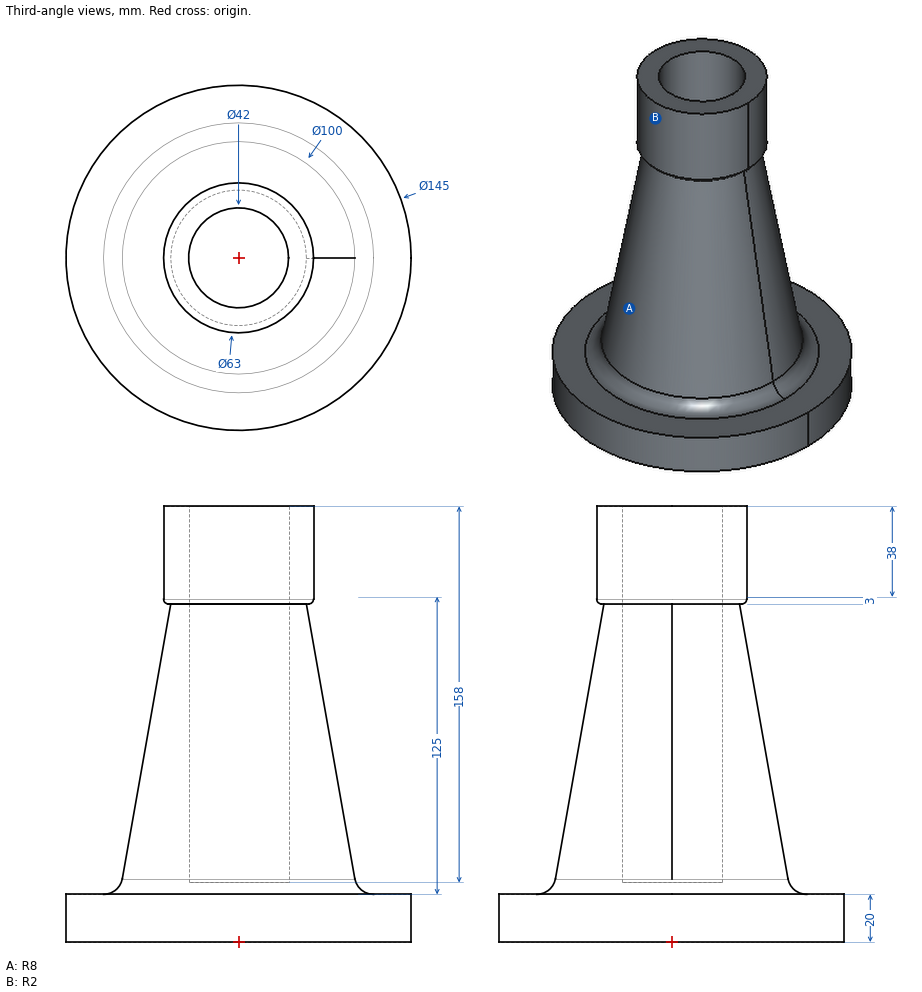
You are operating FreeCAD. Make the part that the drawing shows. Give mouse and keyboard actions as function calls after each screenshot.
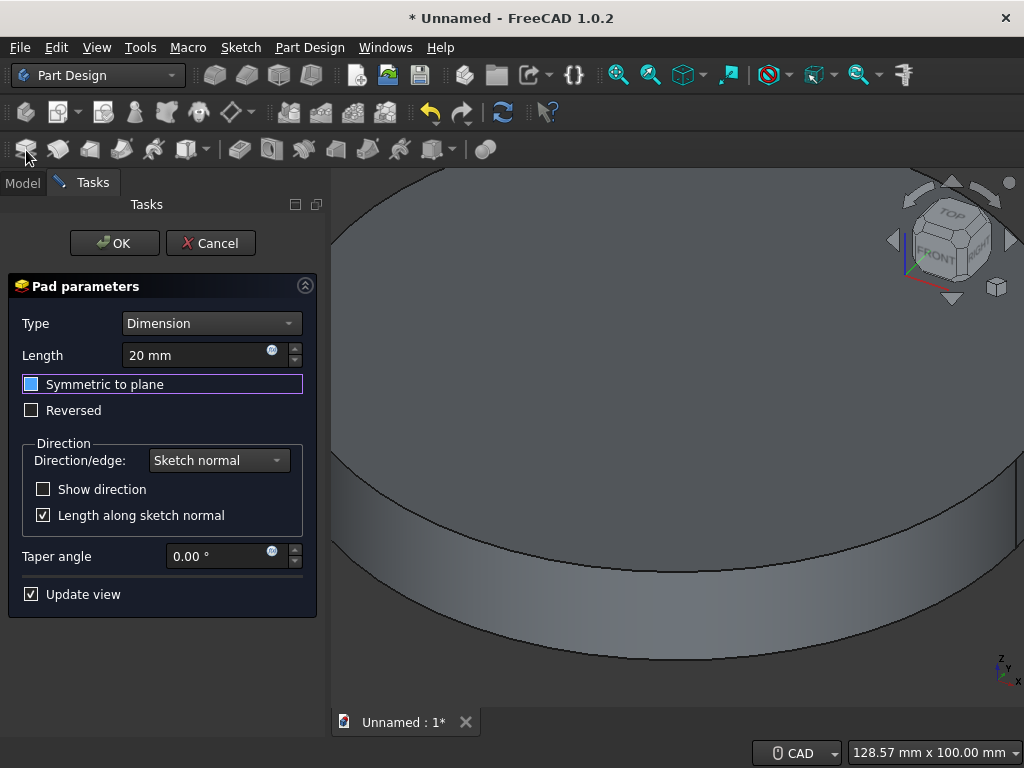
click(115, 243)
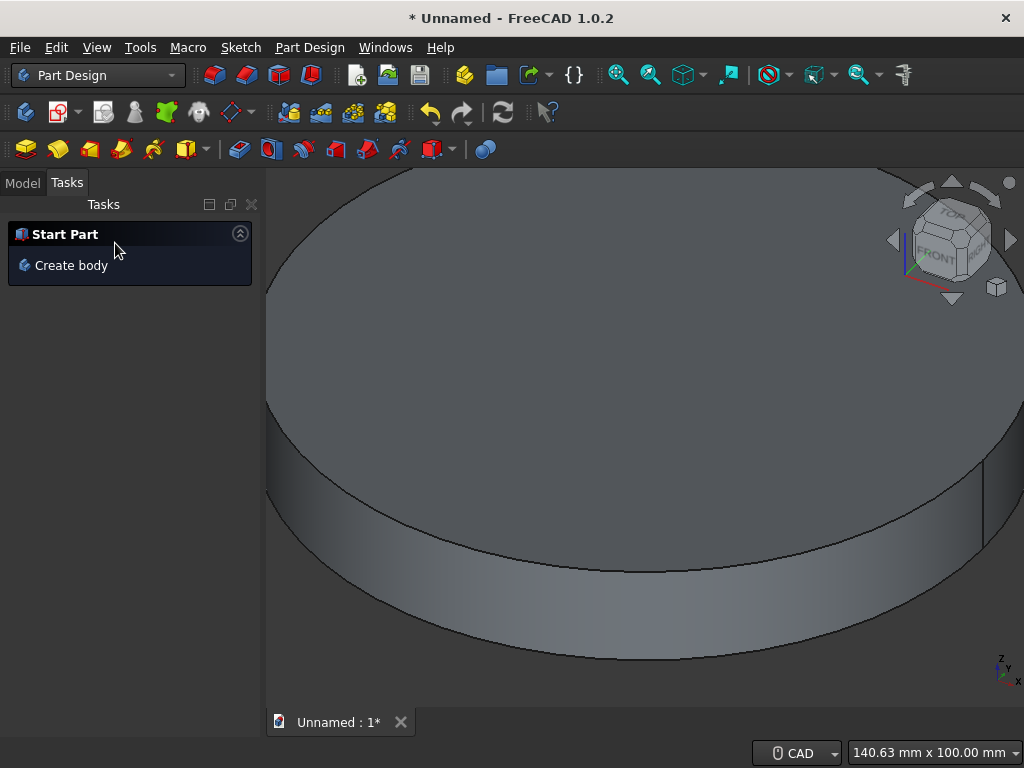
key(v)
key(f)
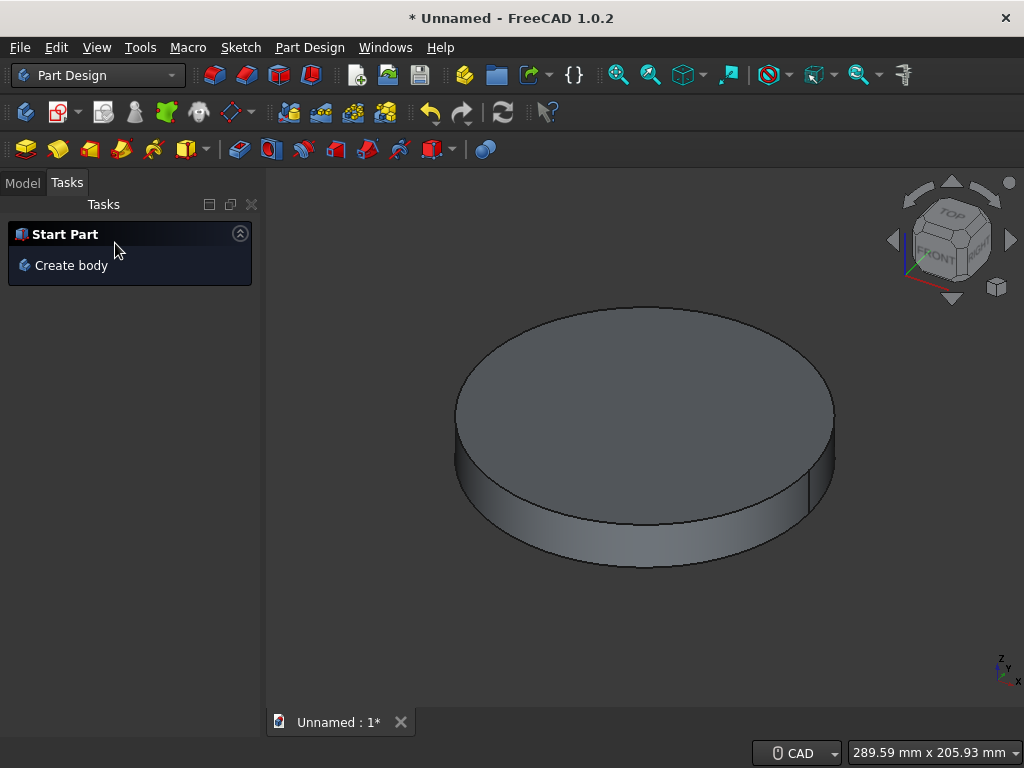
click(645, 415)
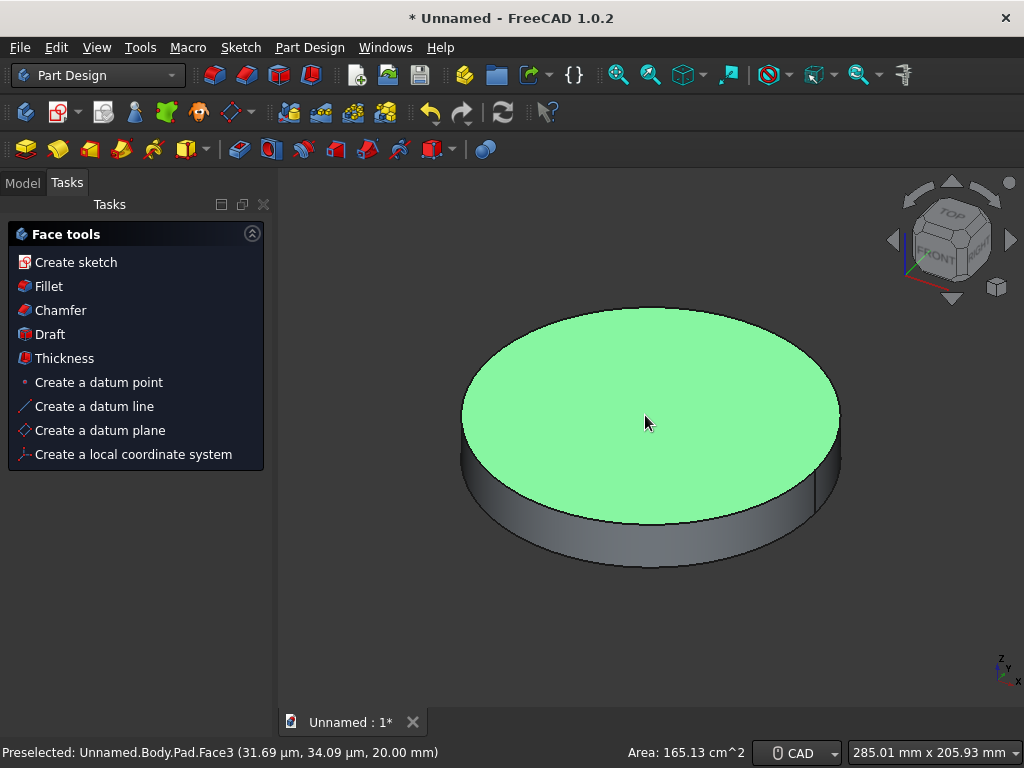
click(58, 112)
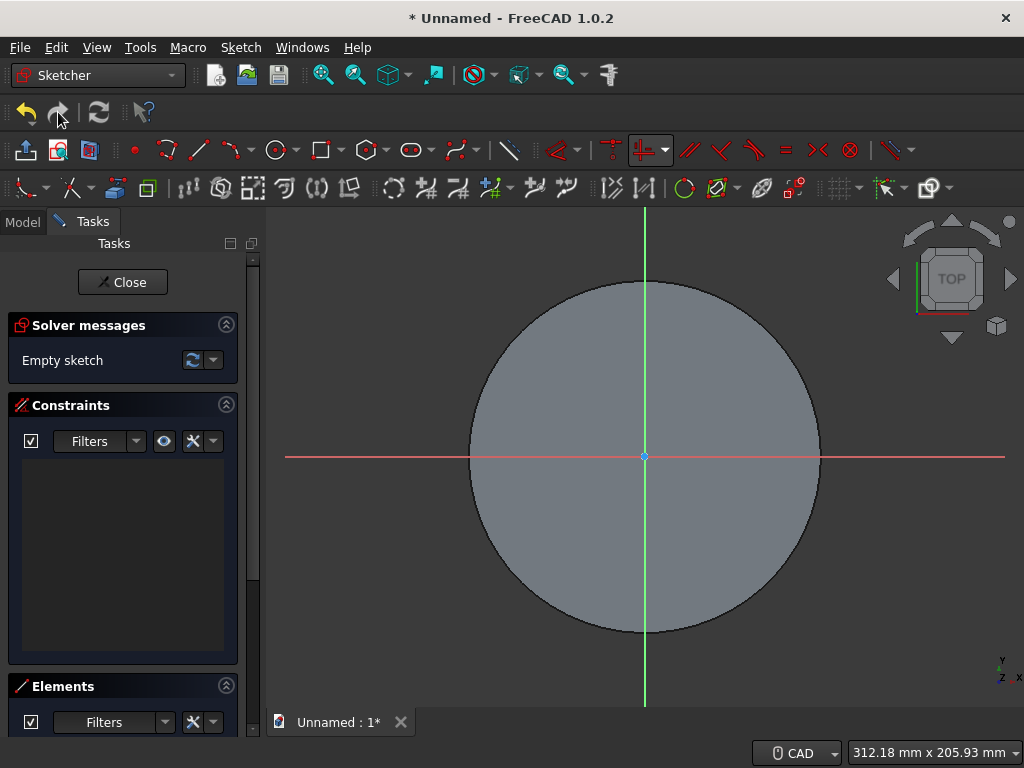
key(g)
key(c)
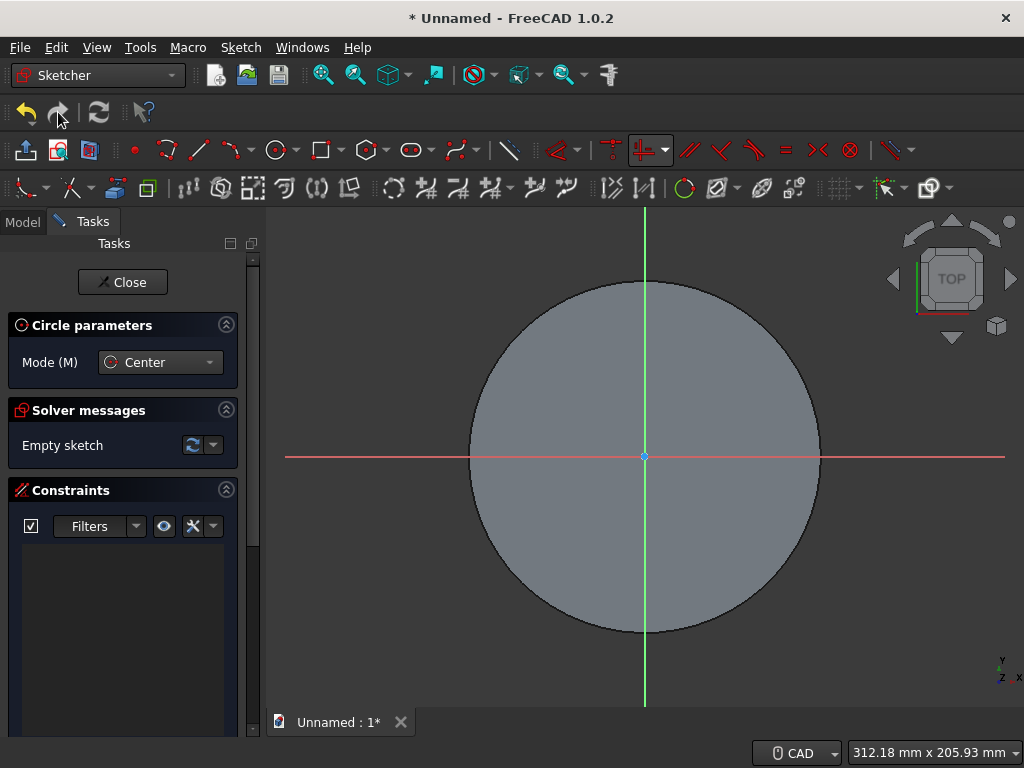
click(645, 457)
click(731, 371)
key(Escape)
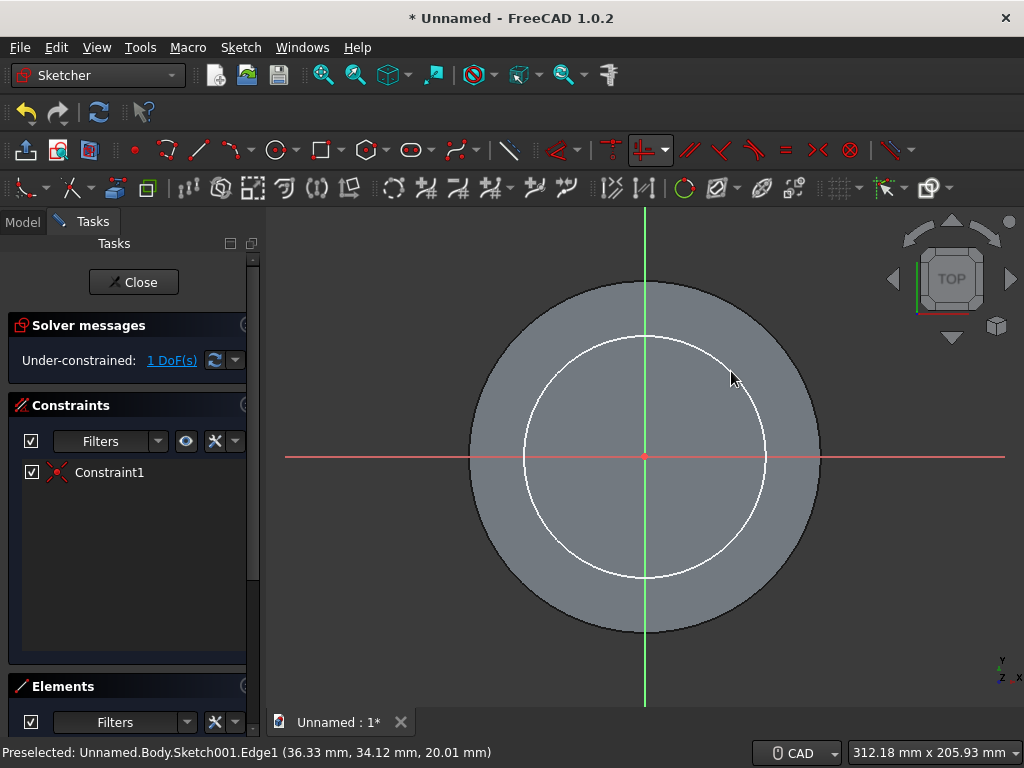
key(d)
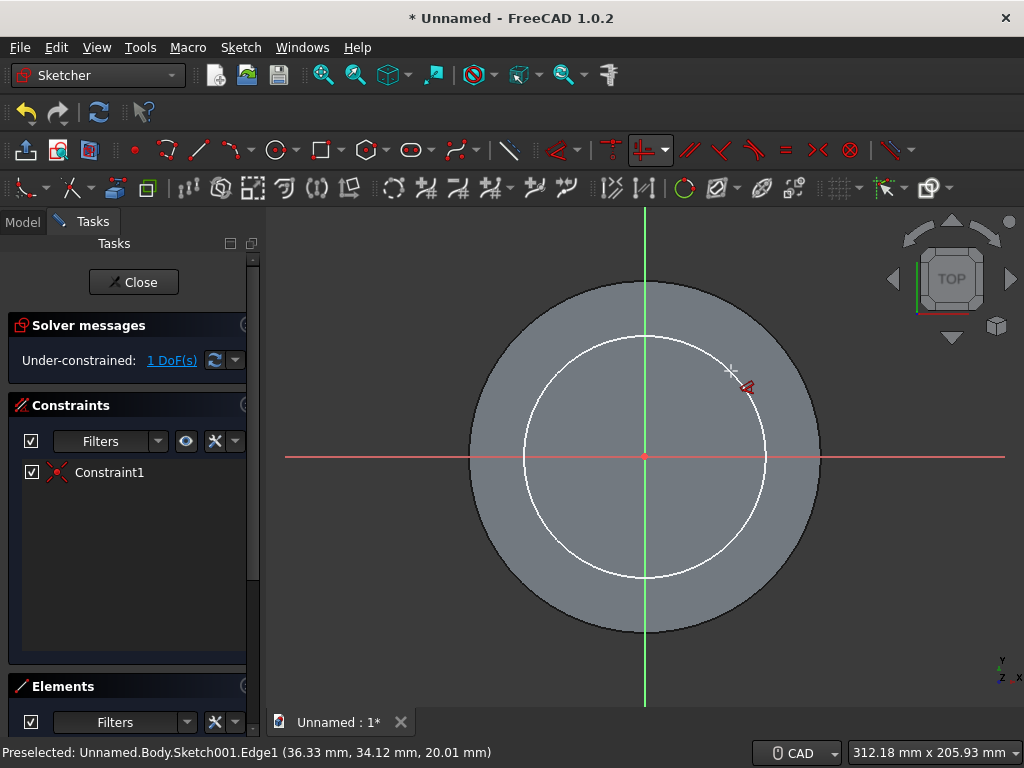
click(730, 371)
click(753, 348)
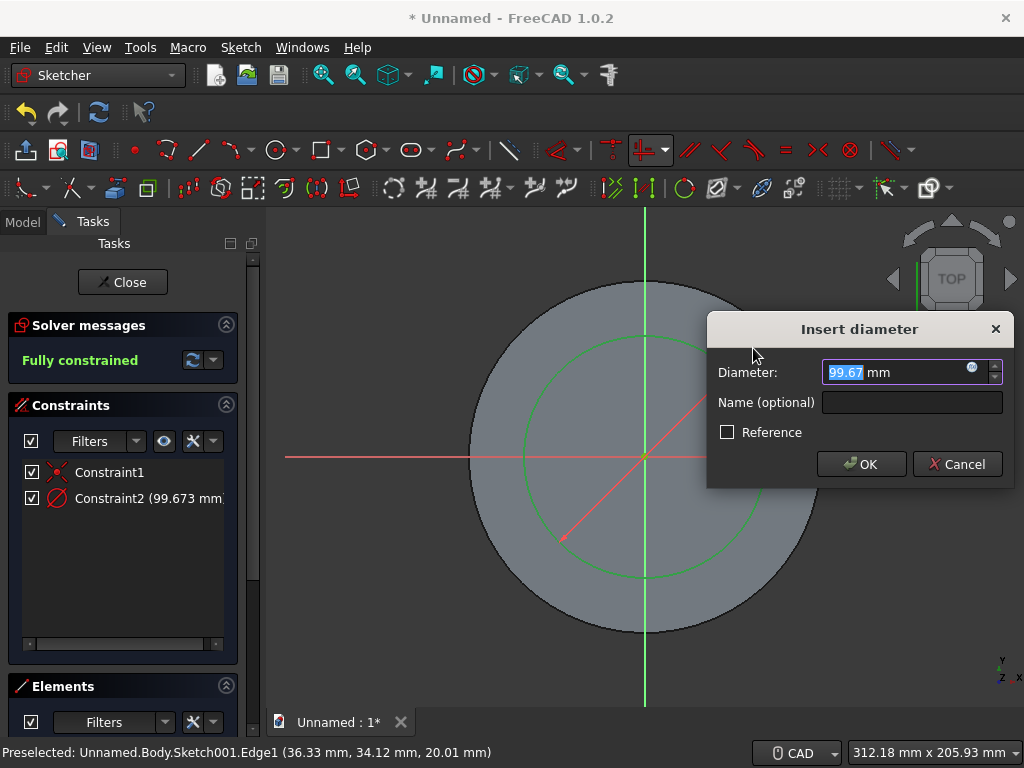
text(100)
key(Return)
key(Escape)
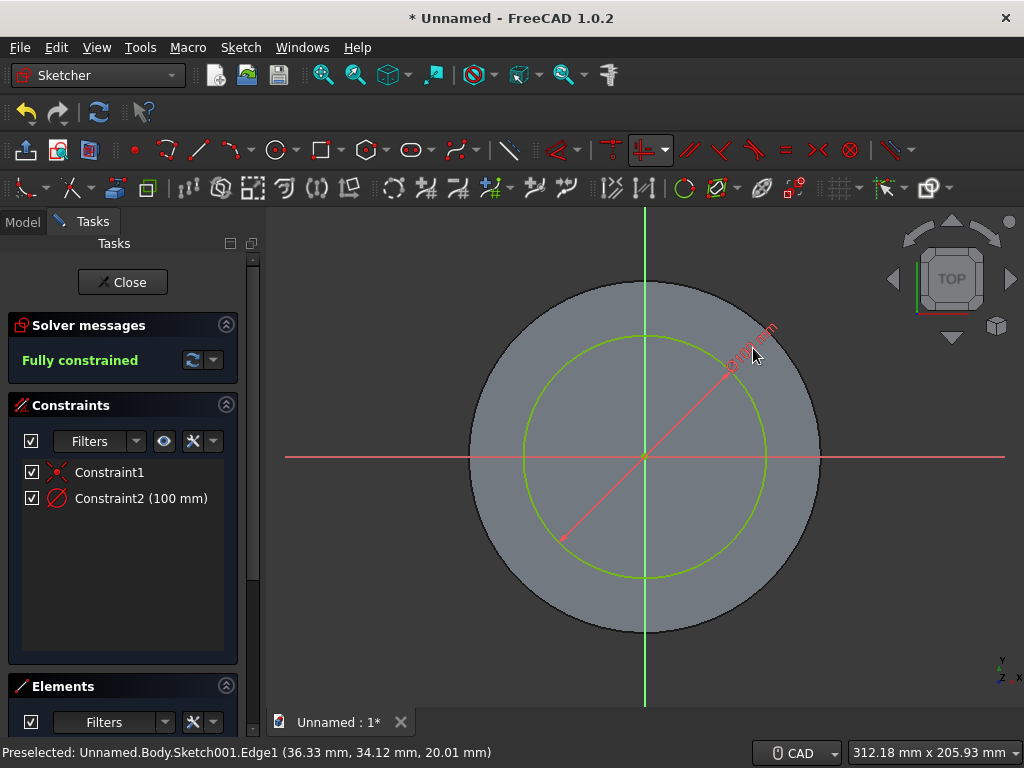
click(123, 282)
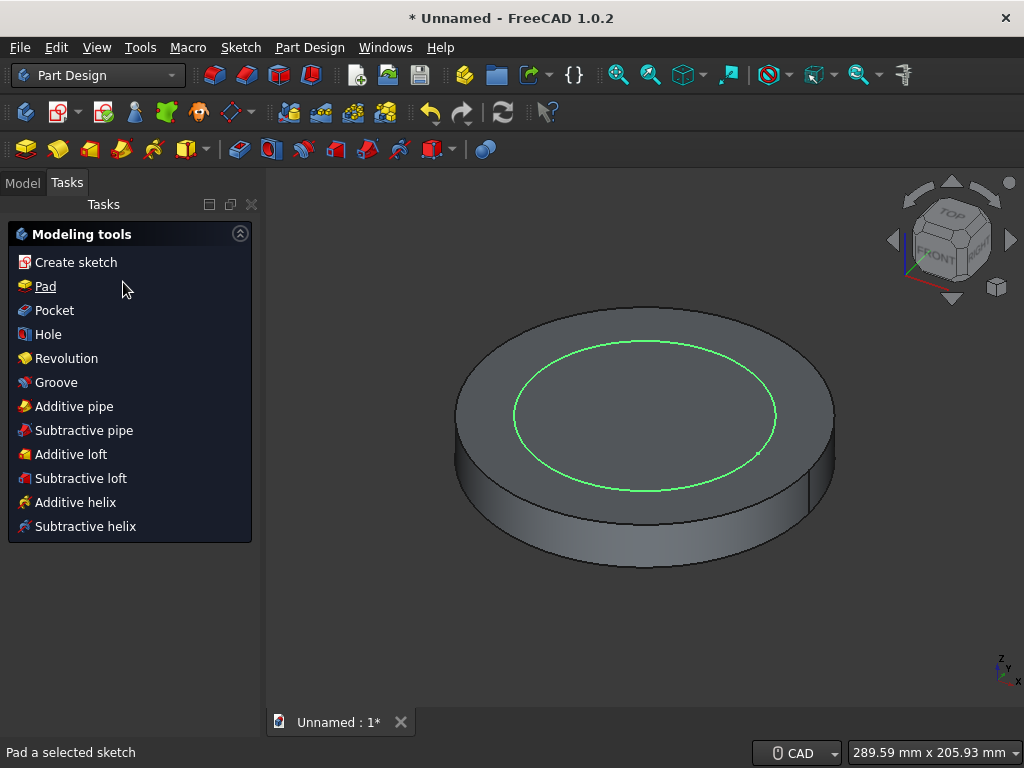
click(26, 150)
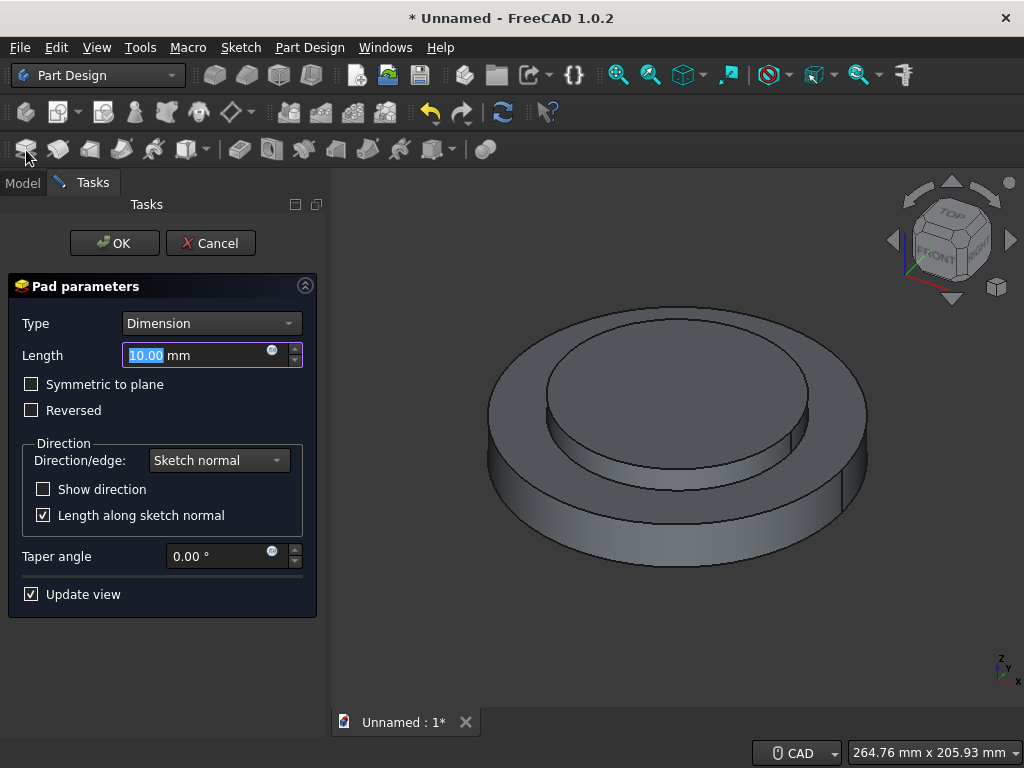
text(125)
key(Tab)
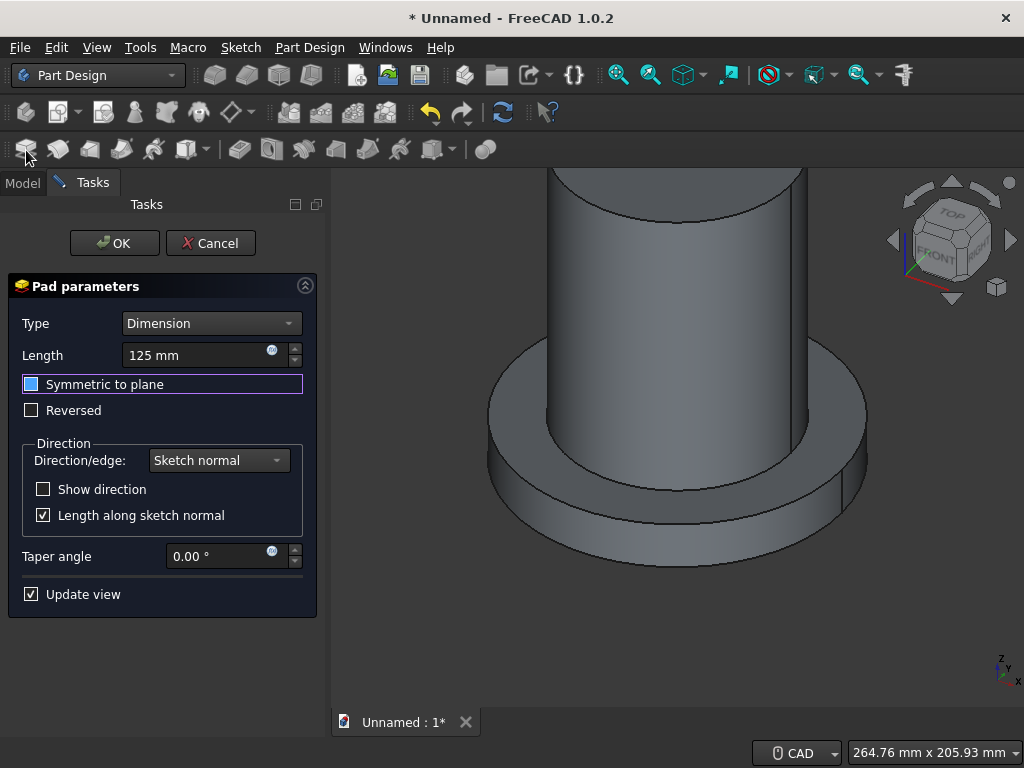
triple_click(226, 556)